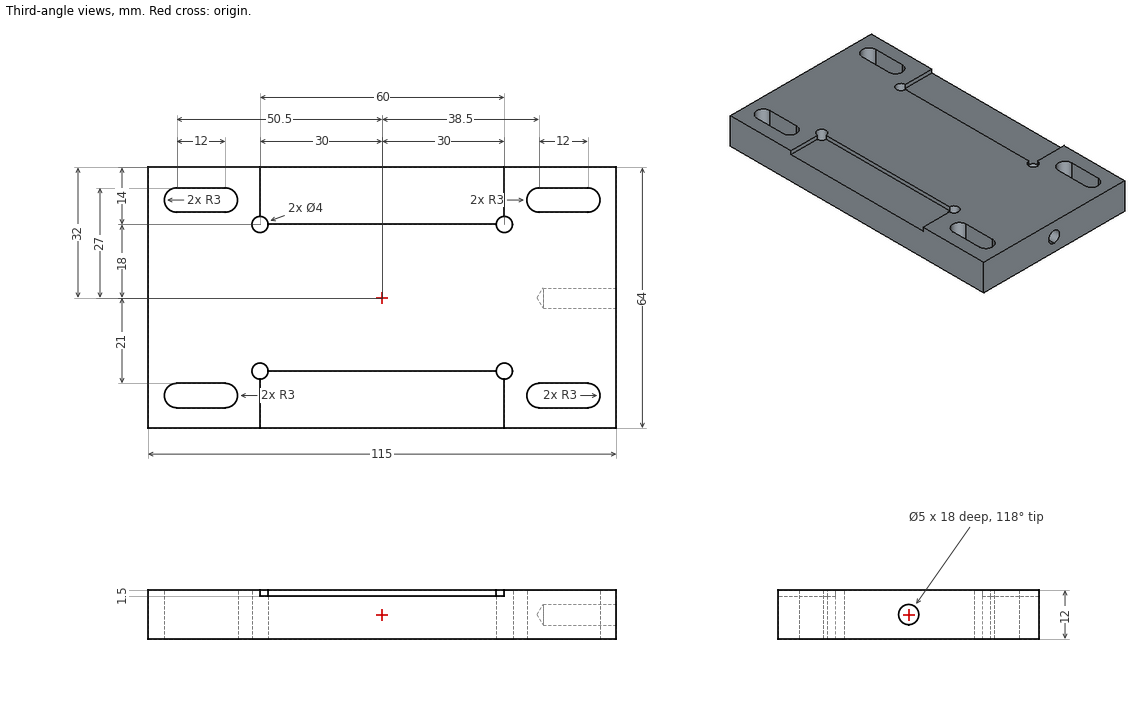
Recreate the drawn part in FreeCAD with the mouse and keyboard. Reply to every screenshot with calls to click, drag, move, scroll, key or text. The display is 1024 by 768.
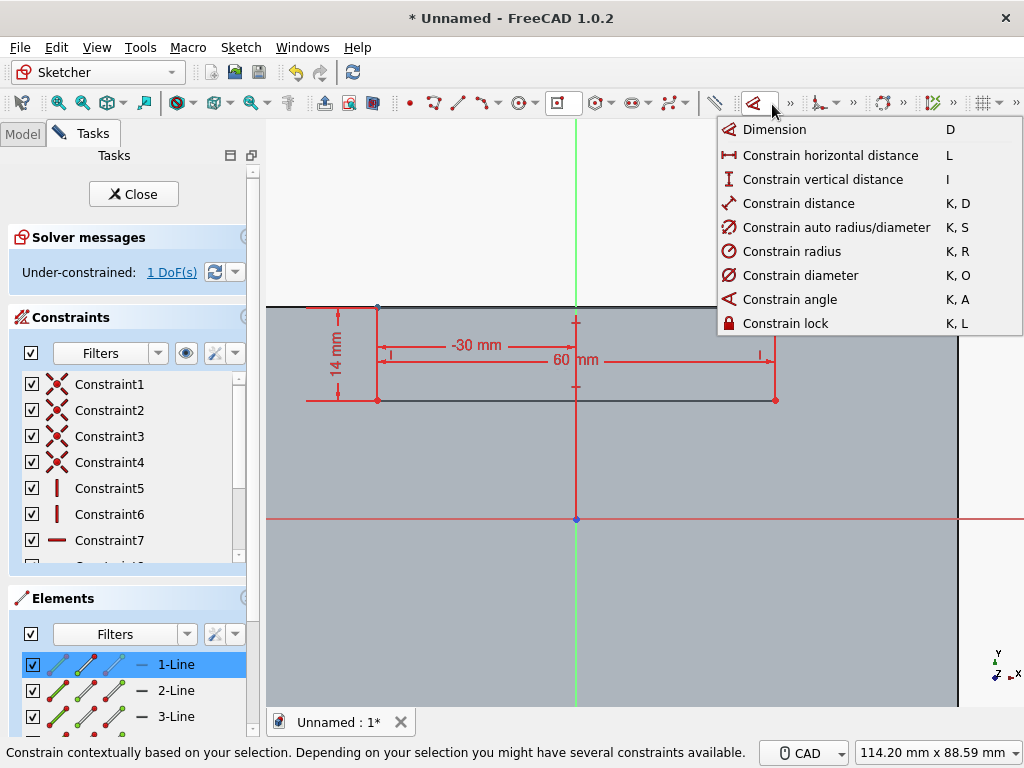
click(870, 179)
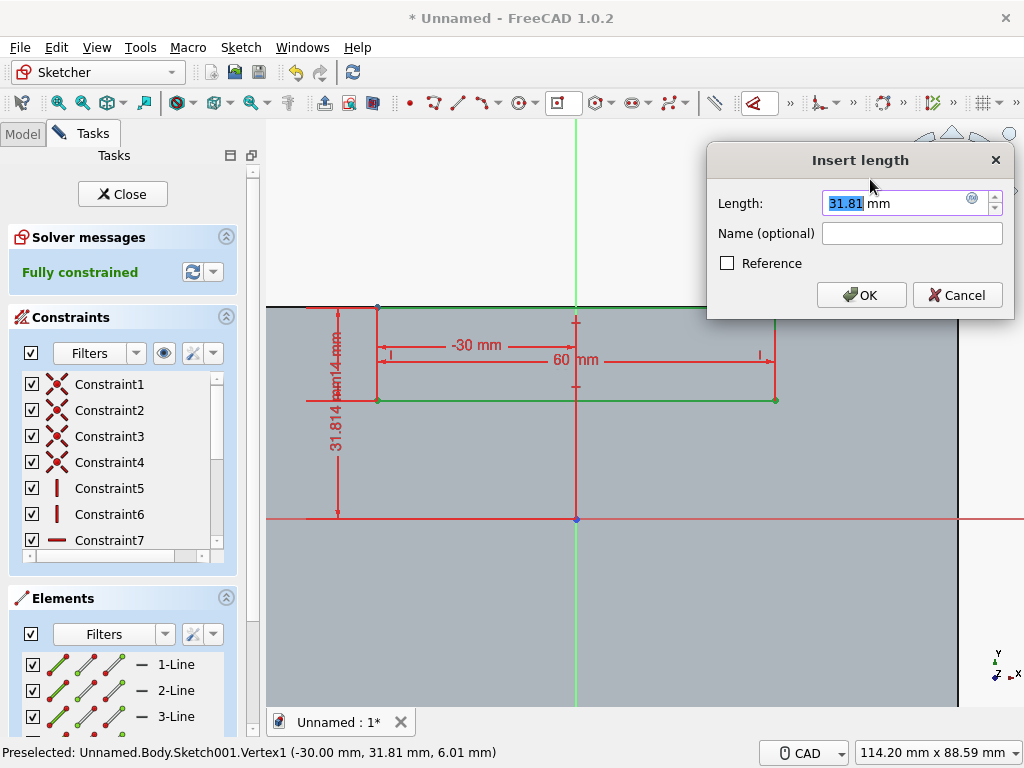
text(32)
key(Return)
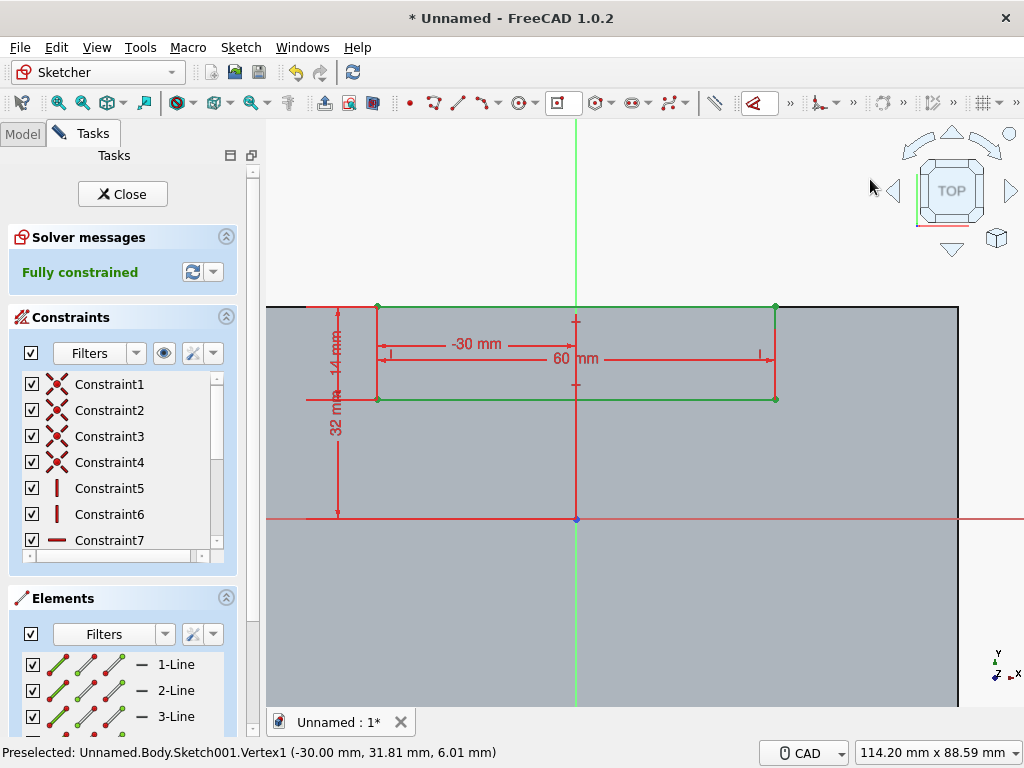
click(123, 194)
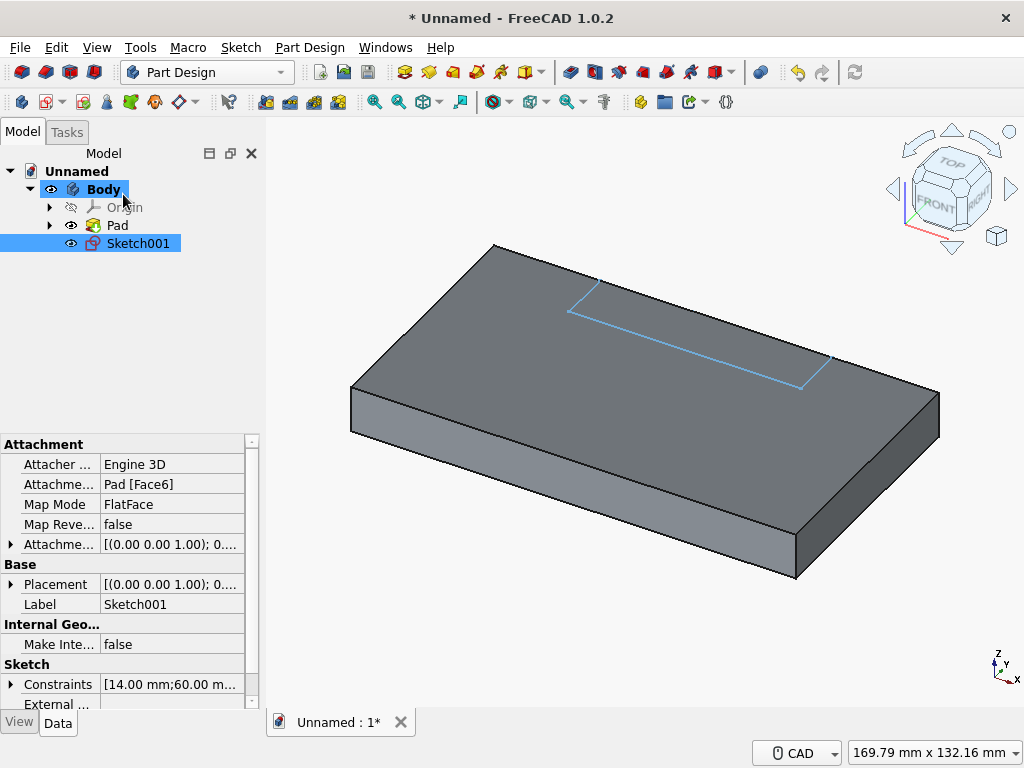
click(572, 72)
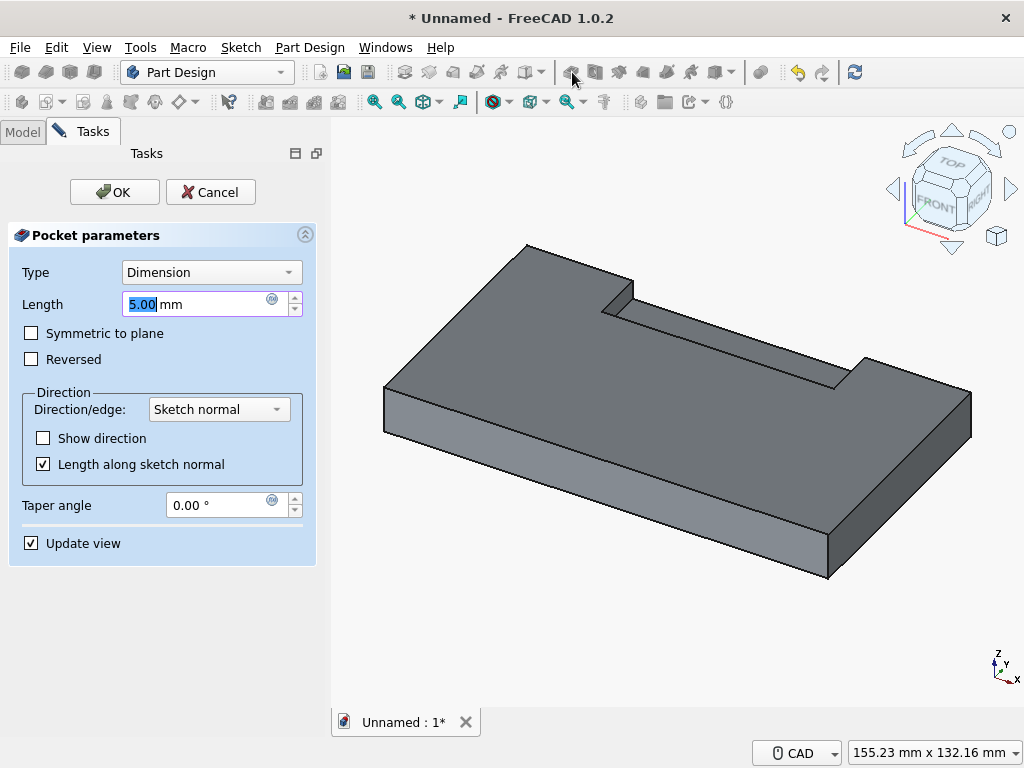
text(1.5)
key(Tab)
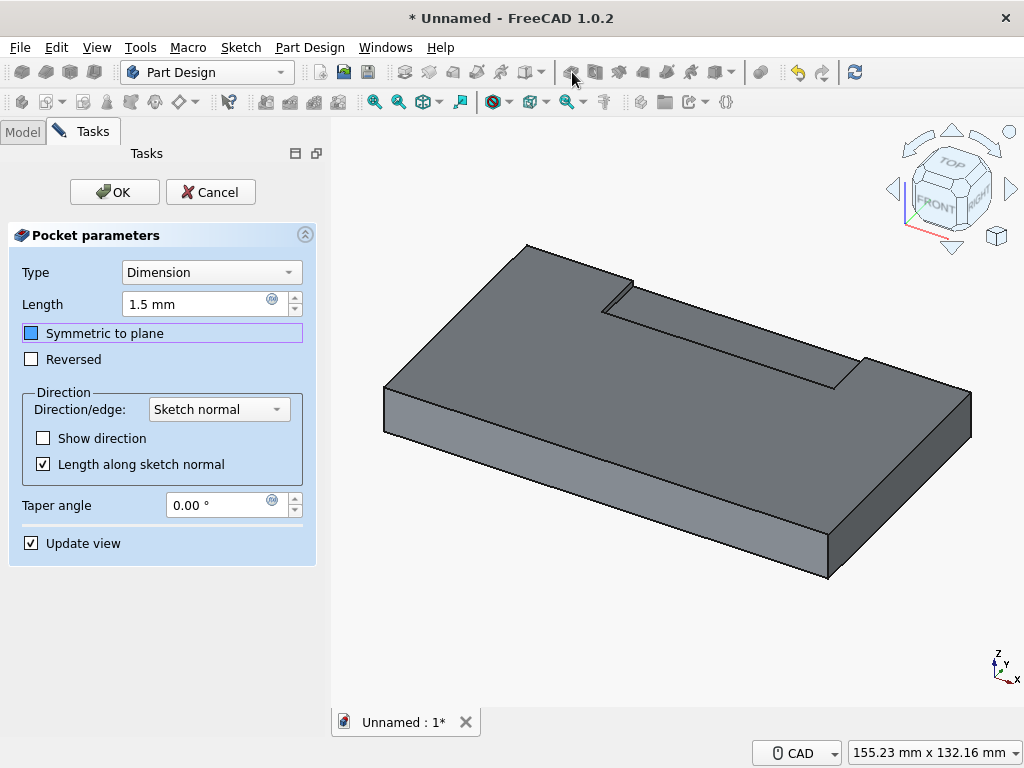
click(115, 192)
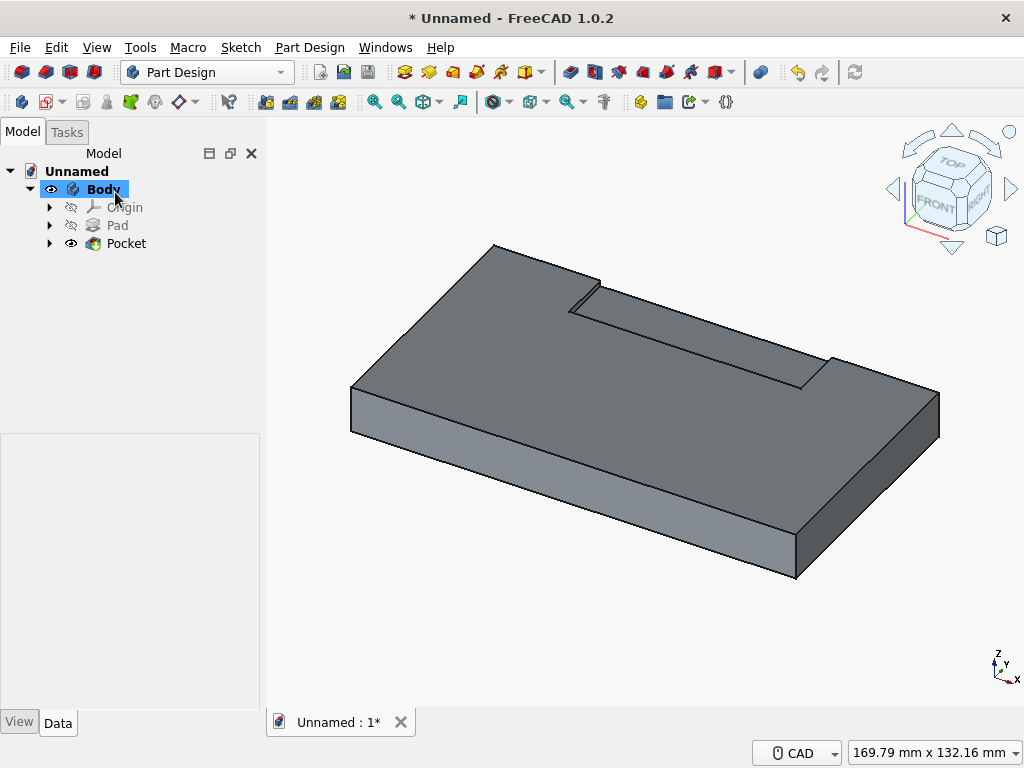
click(752, 451)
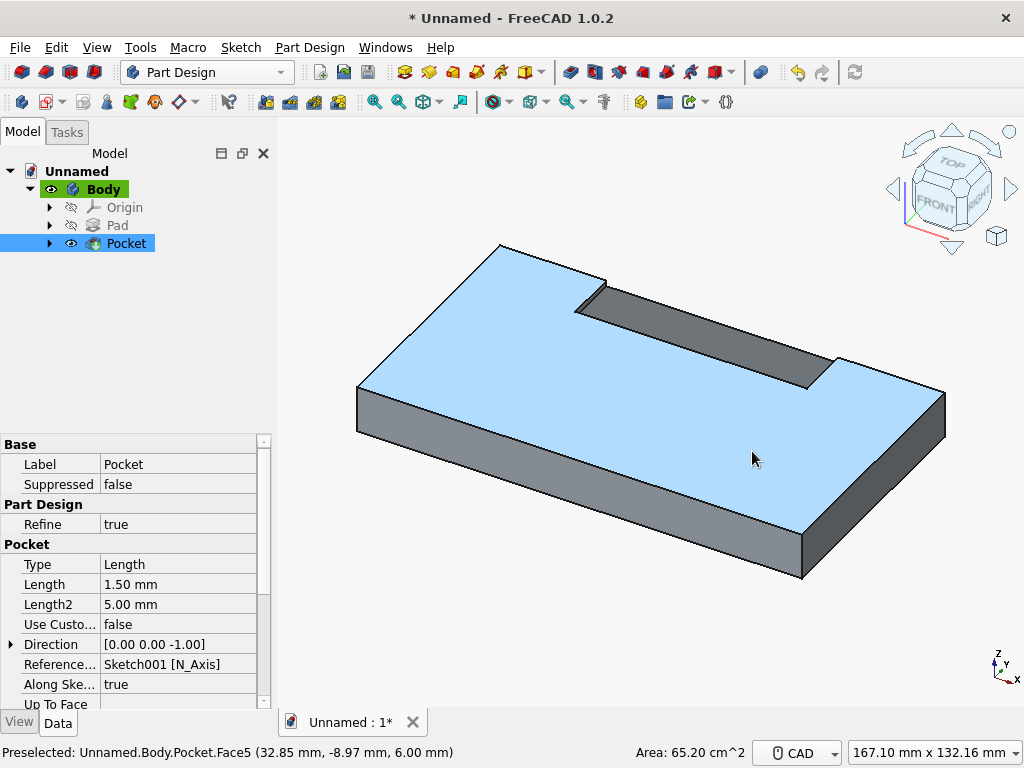
click(46, 102)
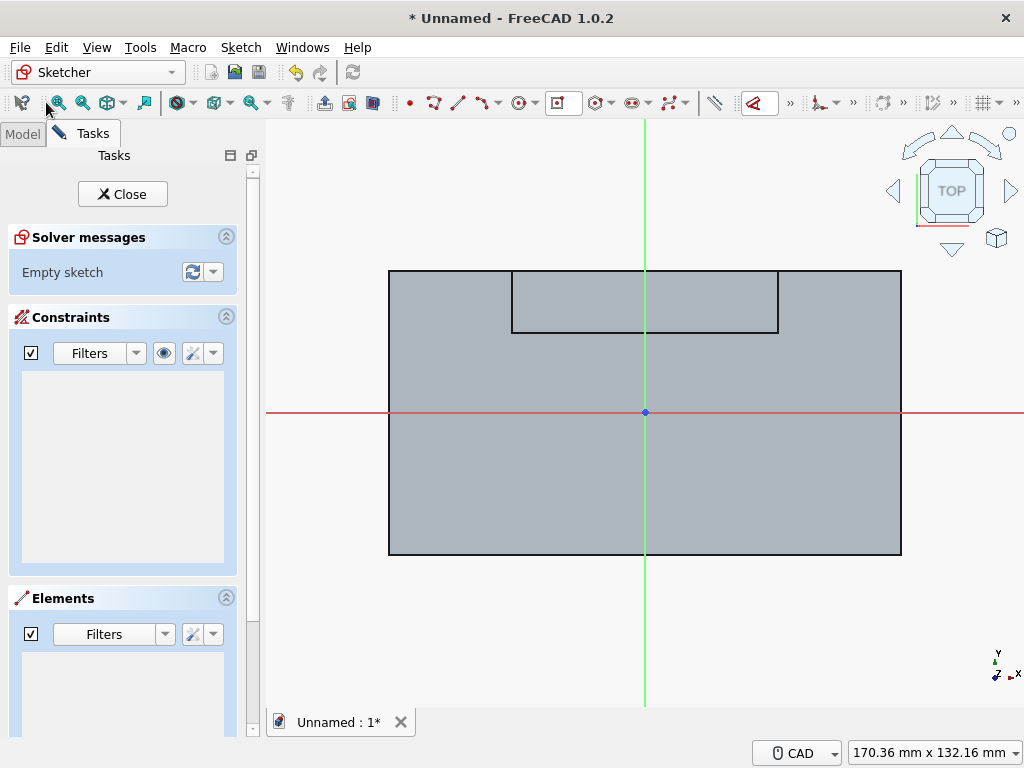
scroll(784, 278, up, 2)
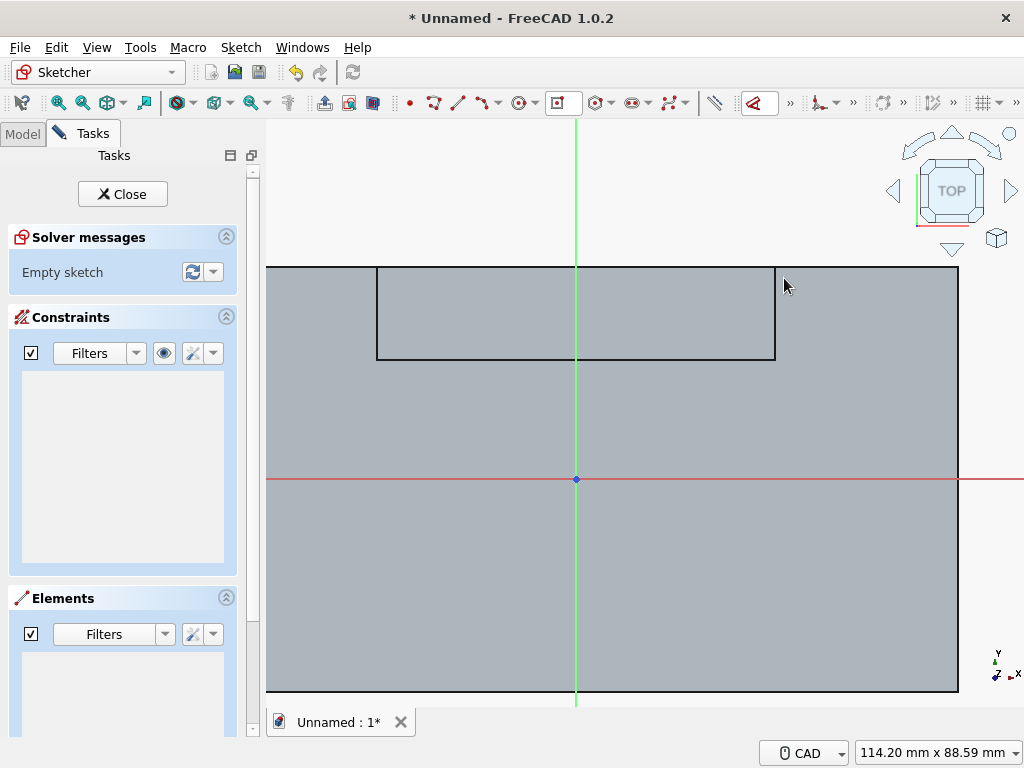
click(520, 104)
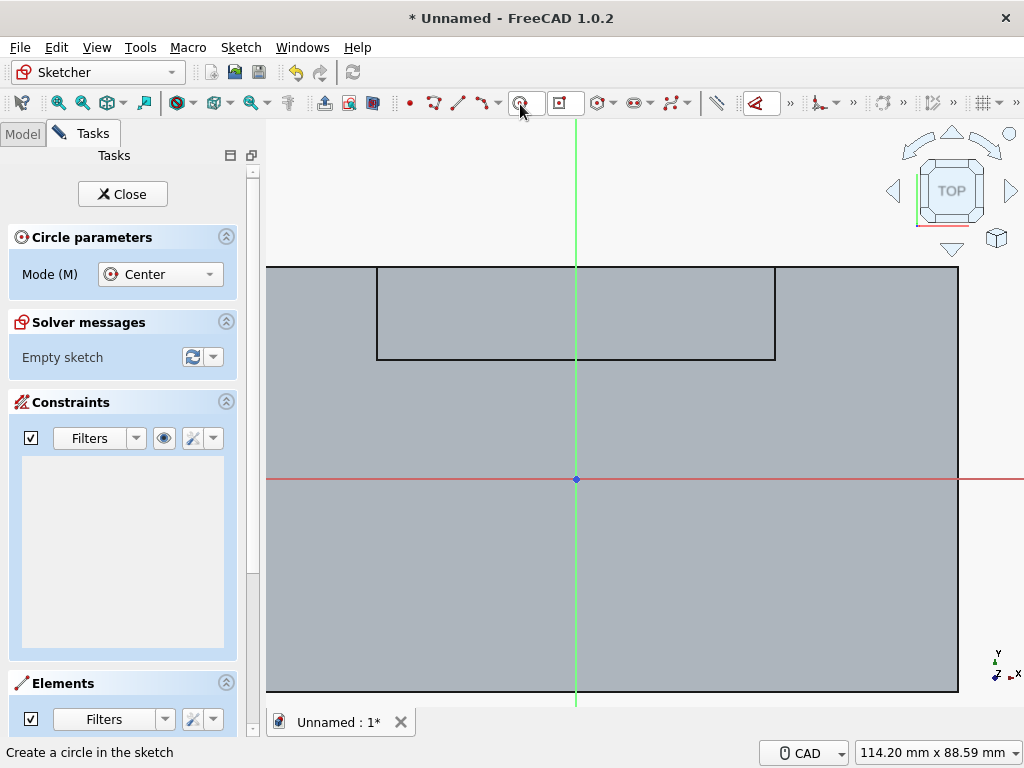
scroll(377, 360, up, 3)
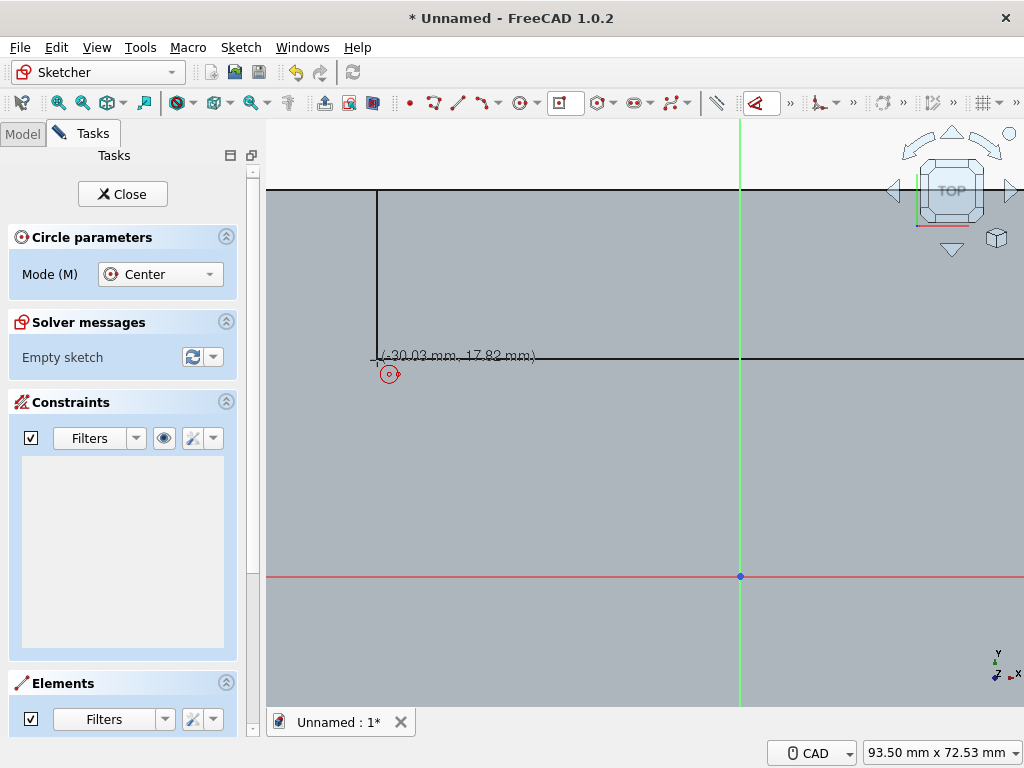
click(377, 359)
click(394, 342)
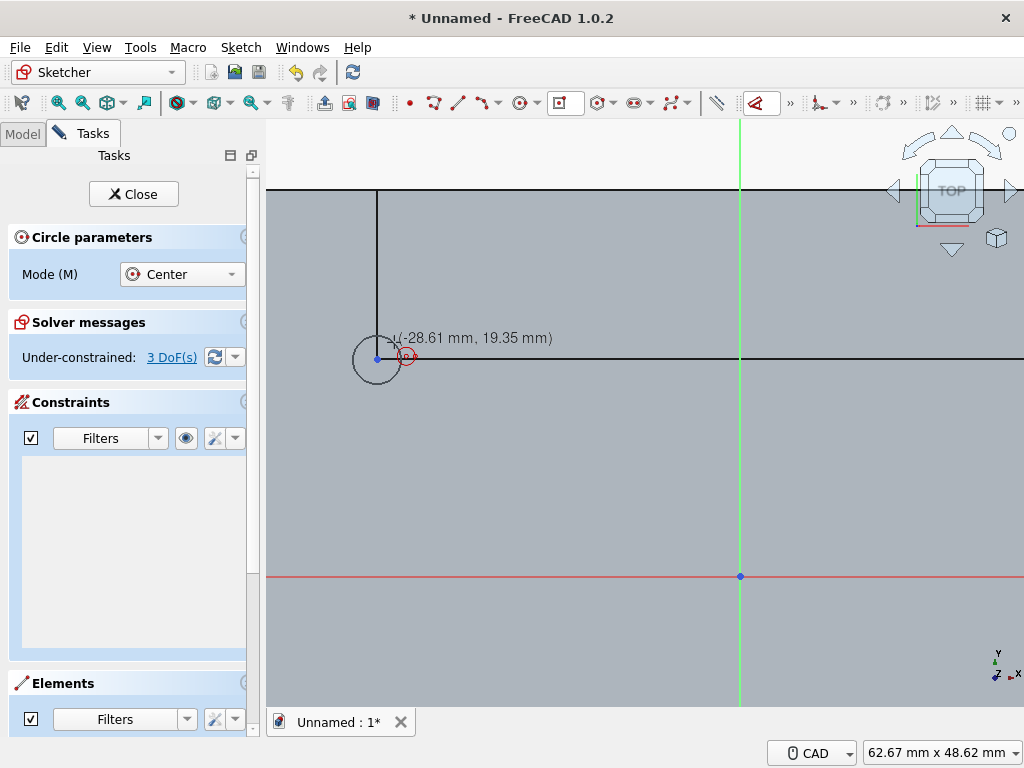
scroll(378, 361, down, 3)